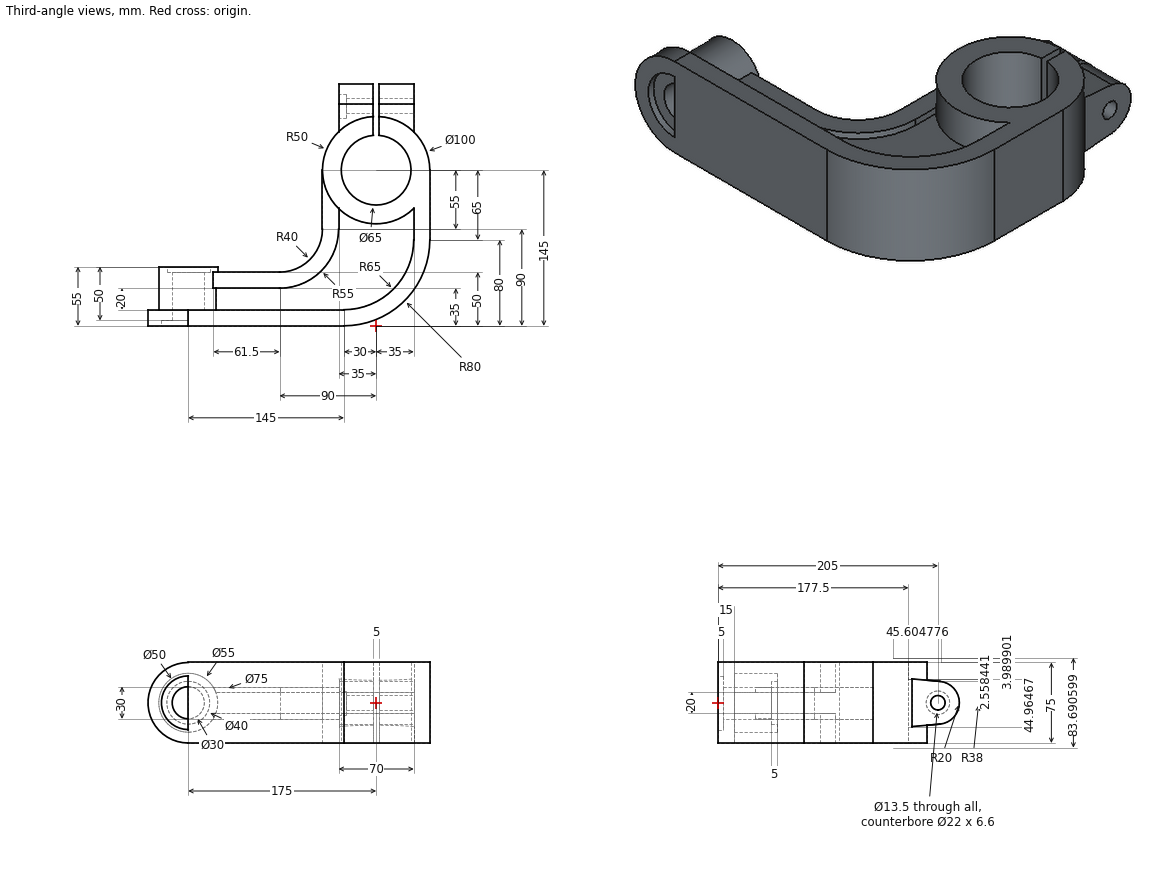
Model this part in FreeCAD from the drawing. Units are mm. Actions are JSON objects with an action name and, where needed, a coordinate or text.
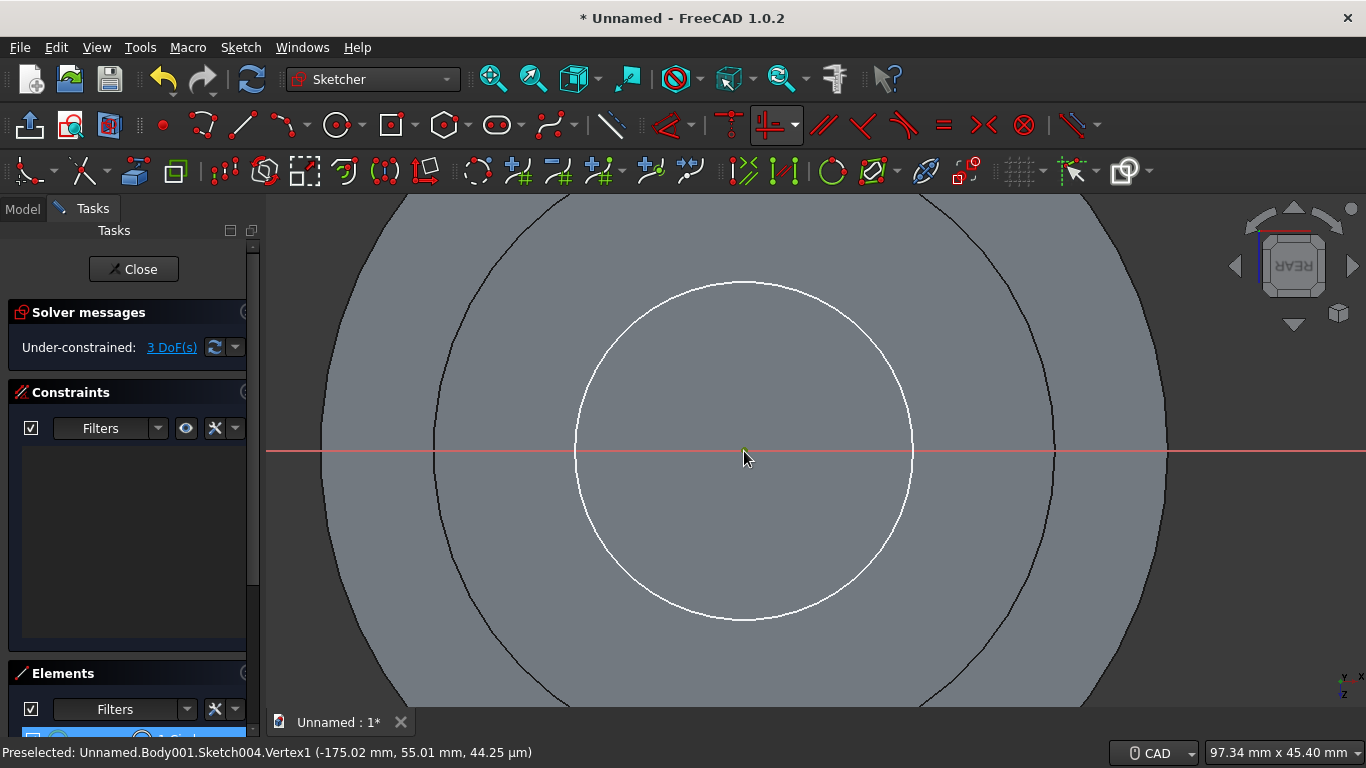
{"action": "left_click", "coordinate": [359, 450]}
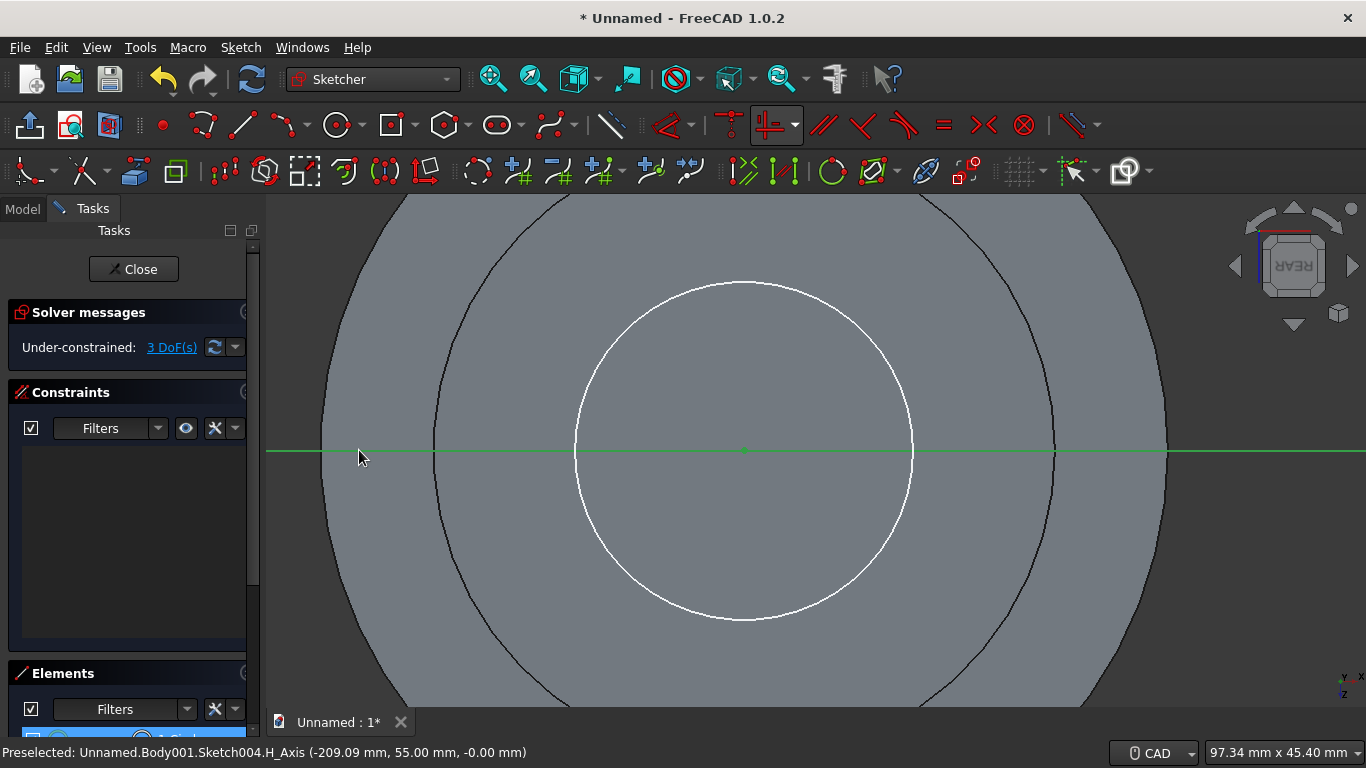
{"action": "key", "text": "c"}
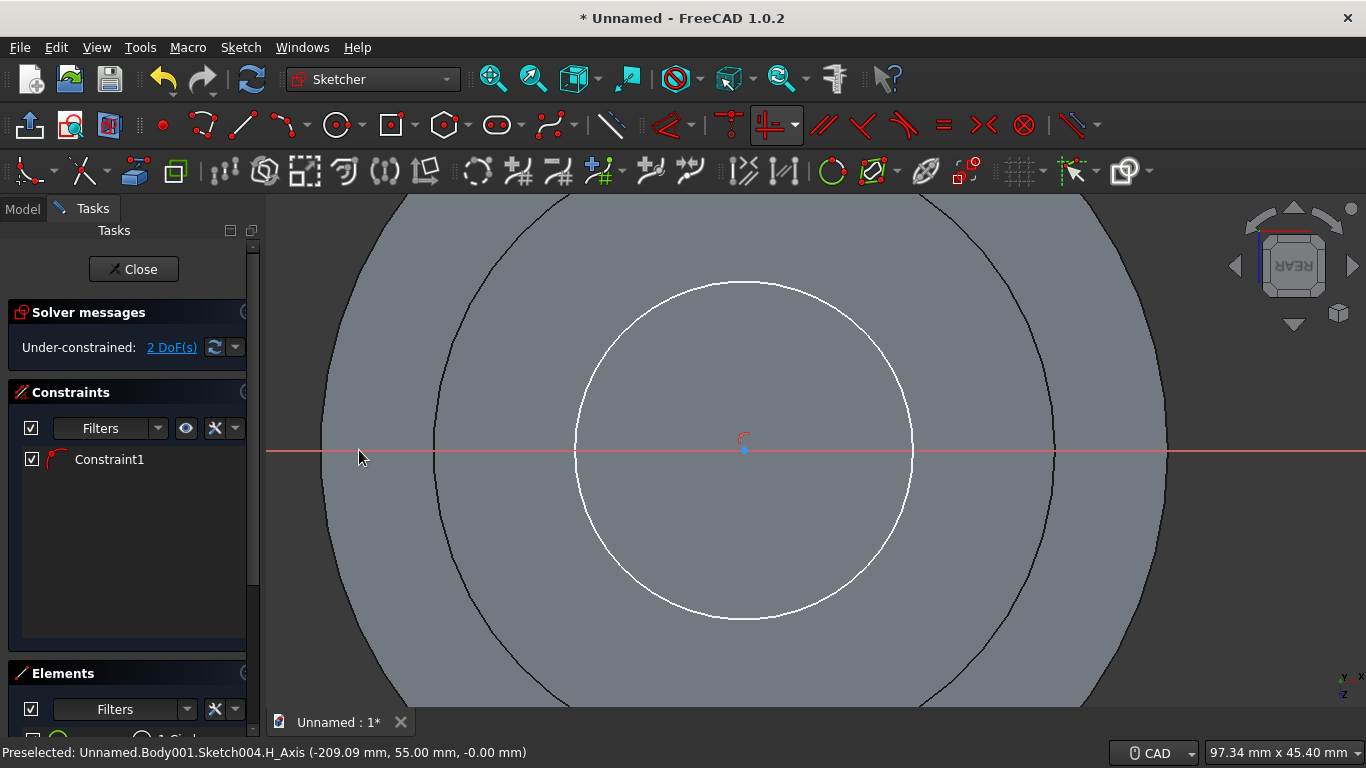
{"action": "left_click", "coordinate": [666, 126]}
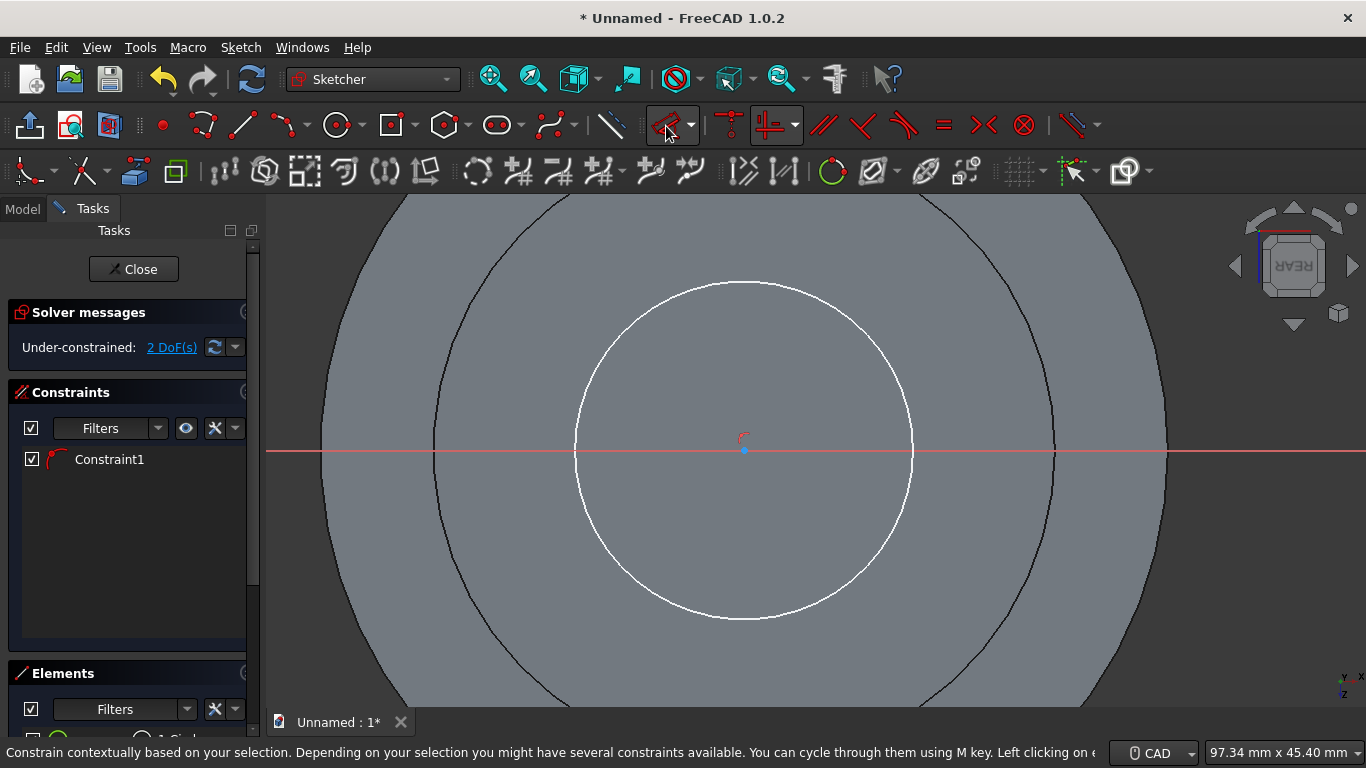
{"action": "left_click", "coordinate": [863, 331]}
{"action": "left_click", "coordinate": [886, 308]}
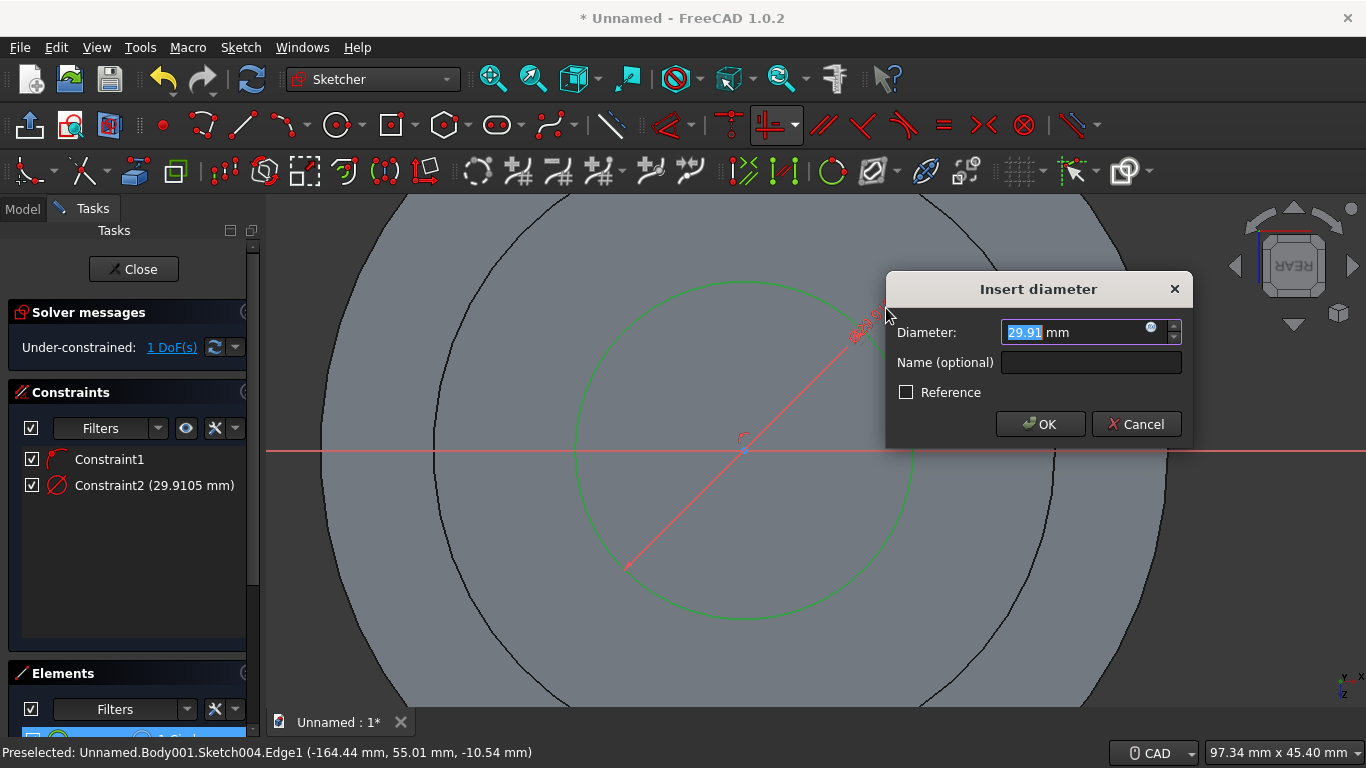
{"action": "type", "text": "30"}
{"action": "key", "text": "Return"}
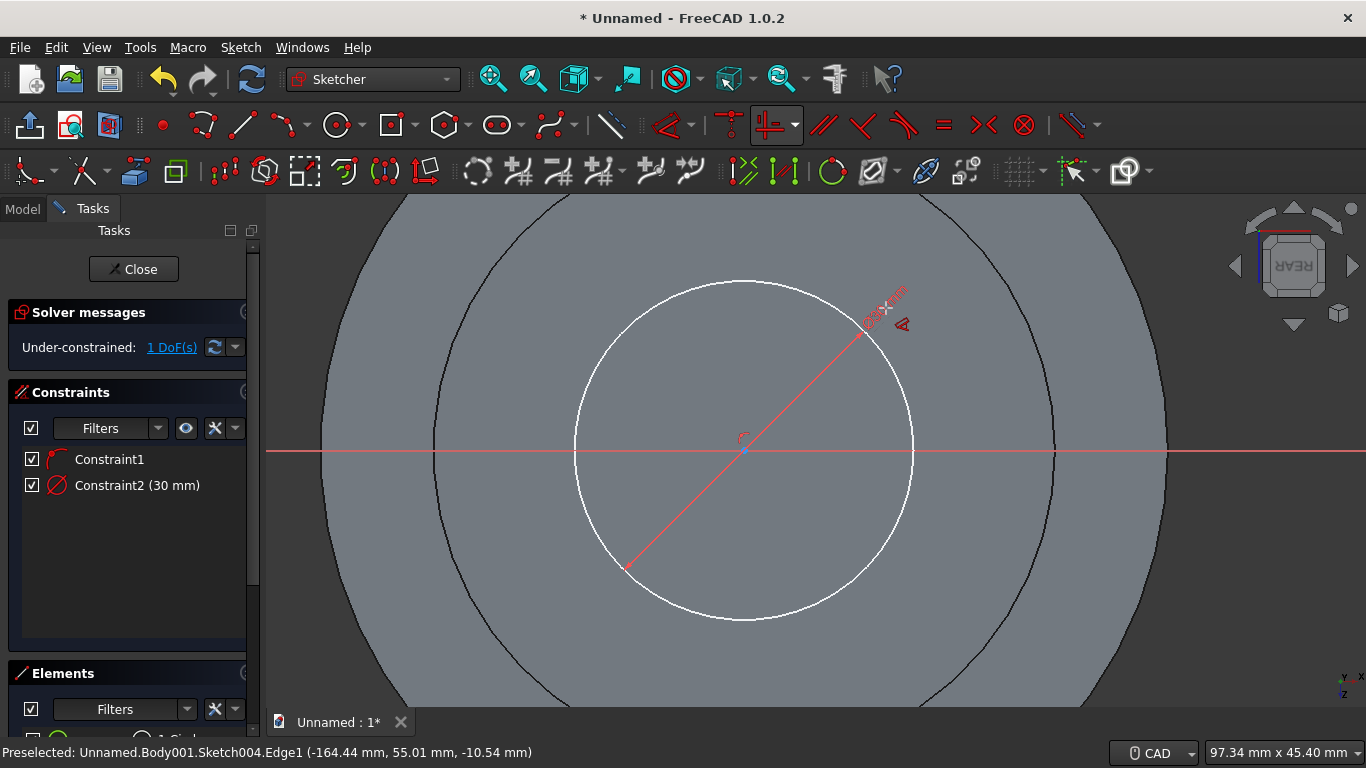
{"action": "left_click", "coordinate": [744, 450]}
{"action": "left_click", "coordinate": [973, 484]}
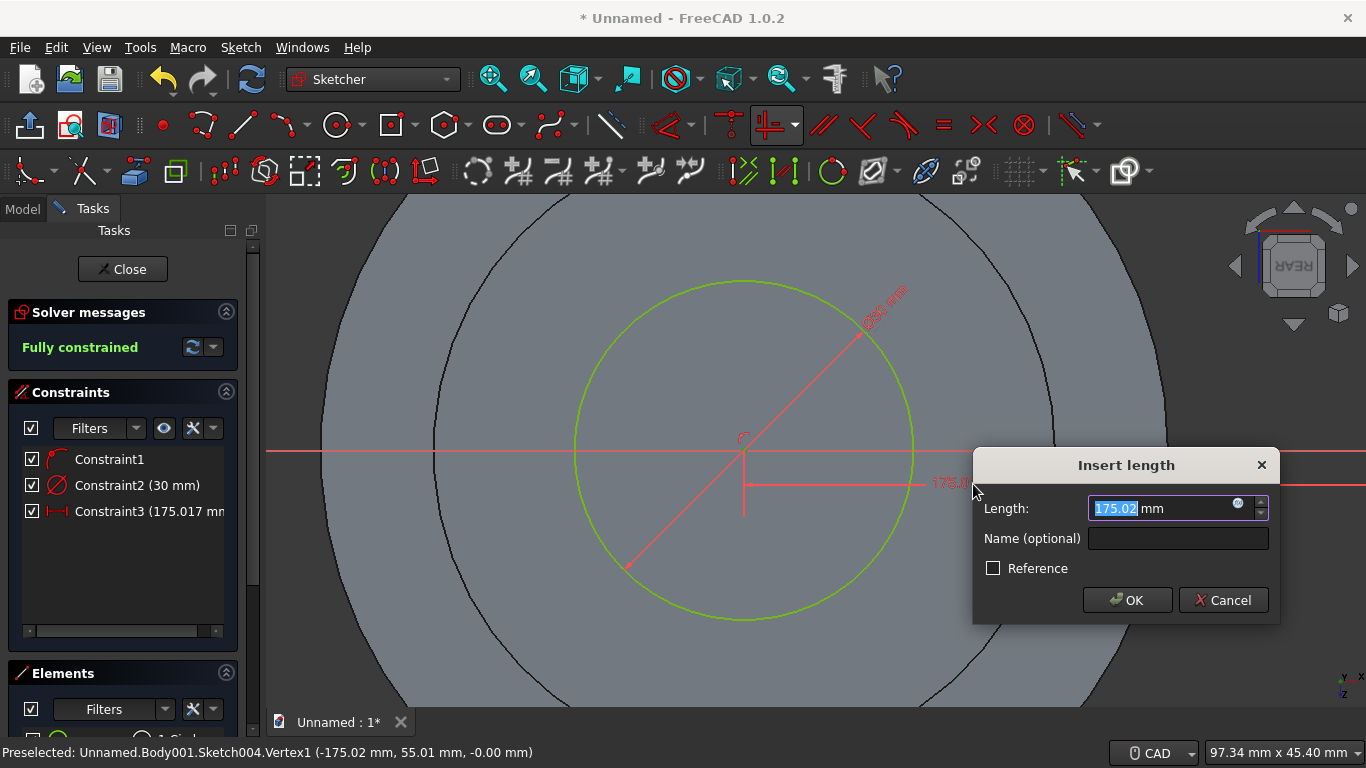
{"action": "type", "text": "175"}
{"action": "key", "text": "Return"}
{"action": "key", "text": "Escape"}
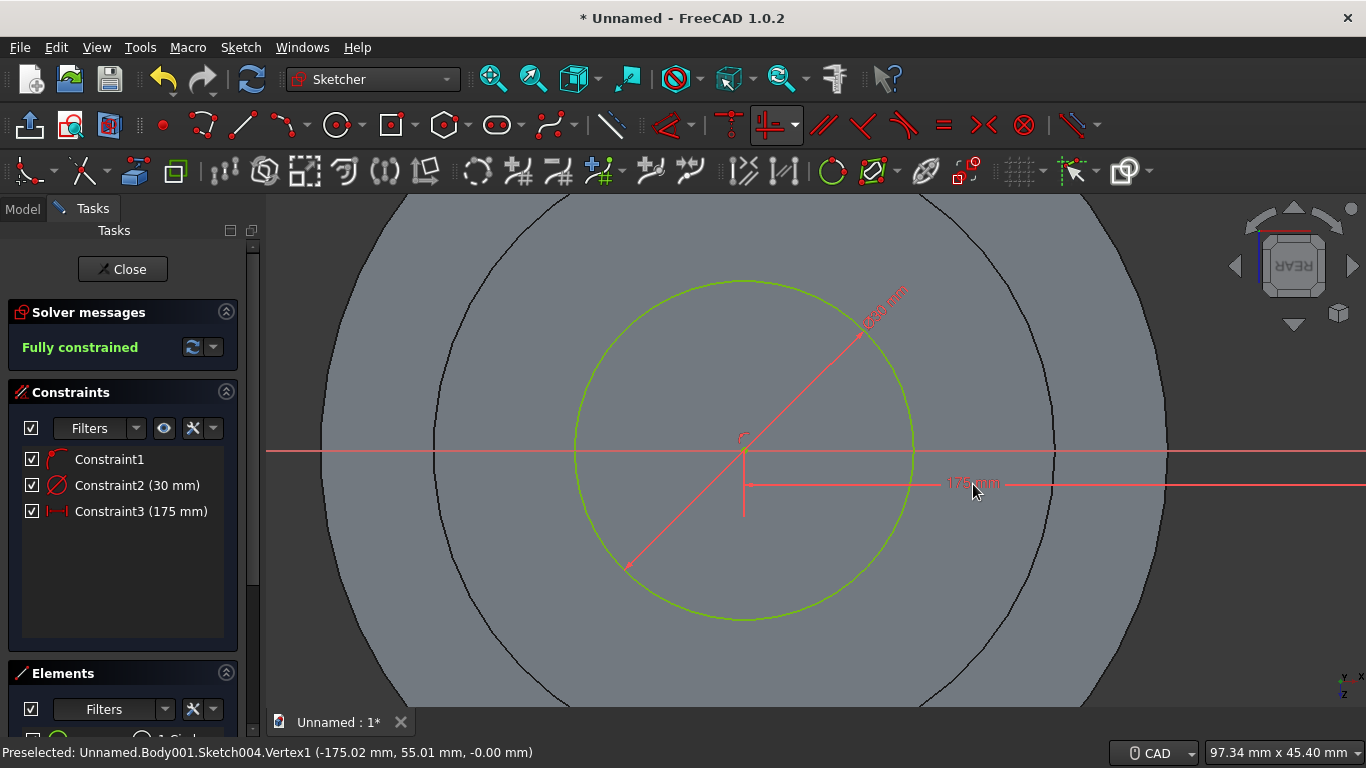
{"action": "left_click", "coordinate": [123, 269]}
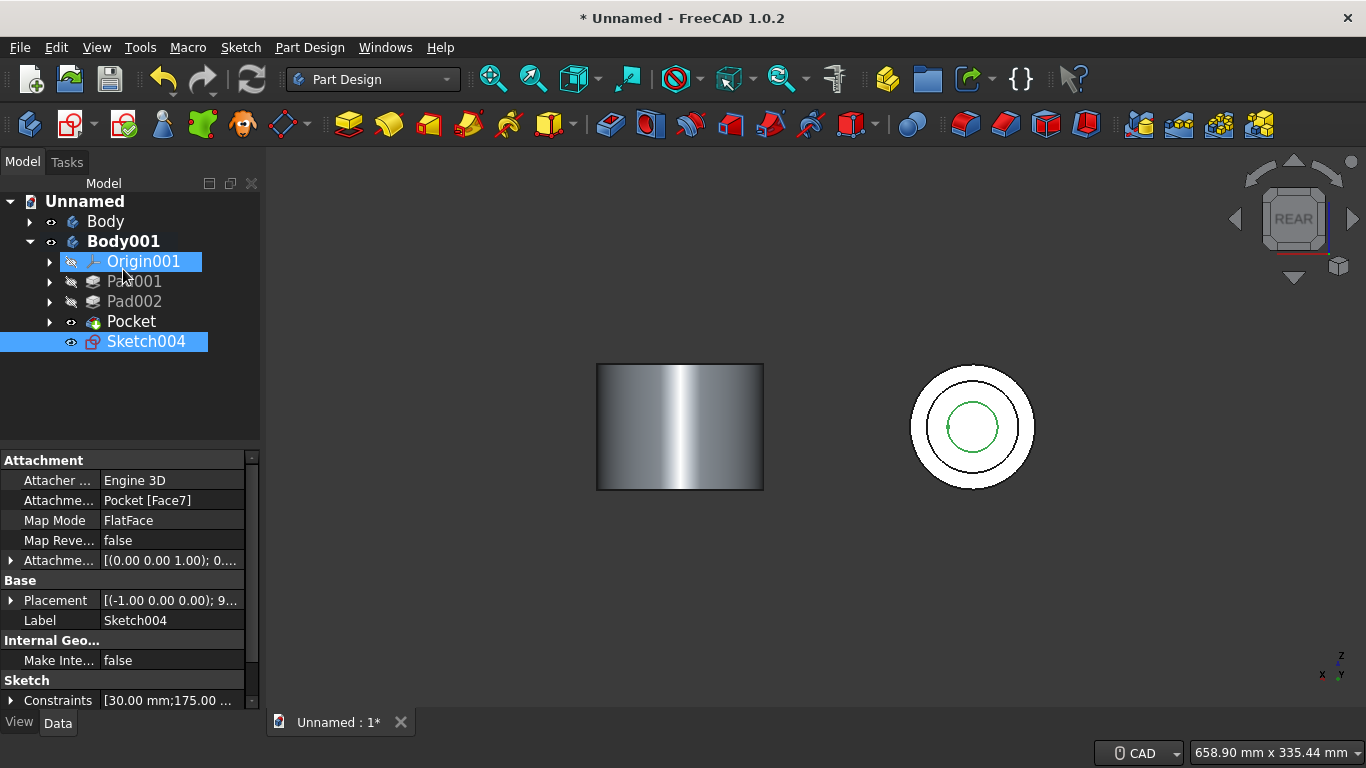
{"action": "left_click", "coordinate": [612, 124]}